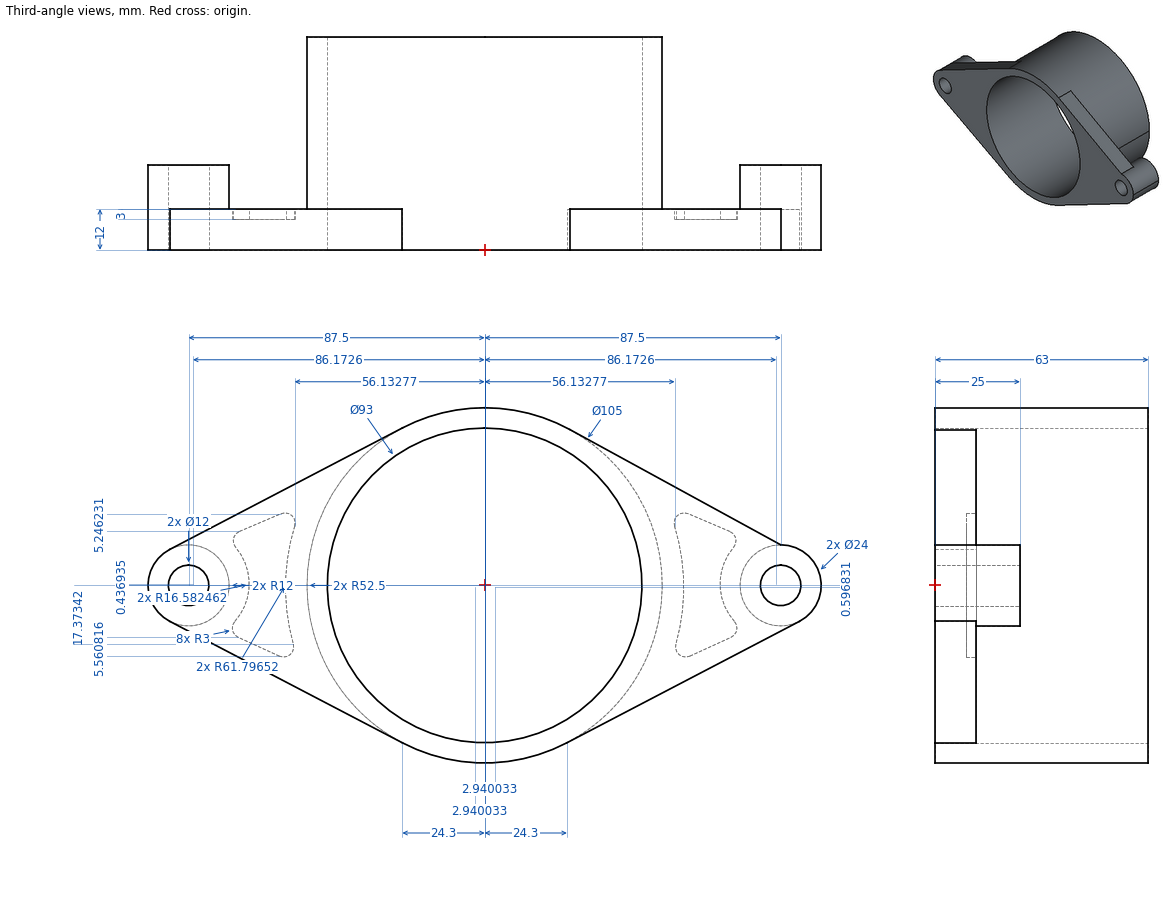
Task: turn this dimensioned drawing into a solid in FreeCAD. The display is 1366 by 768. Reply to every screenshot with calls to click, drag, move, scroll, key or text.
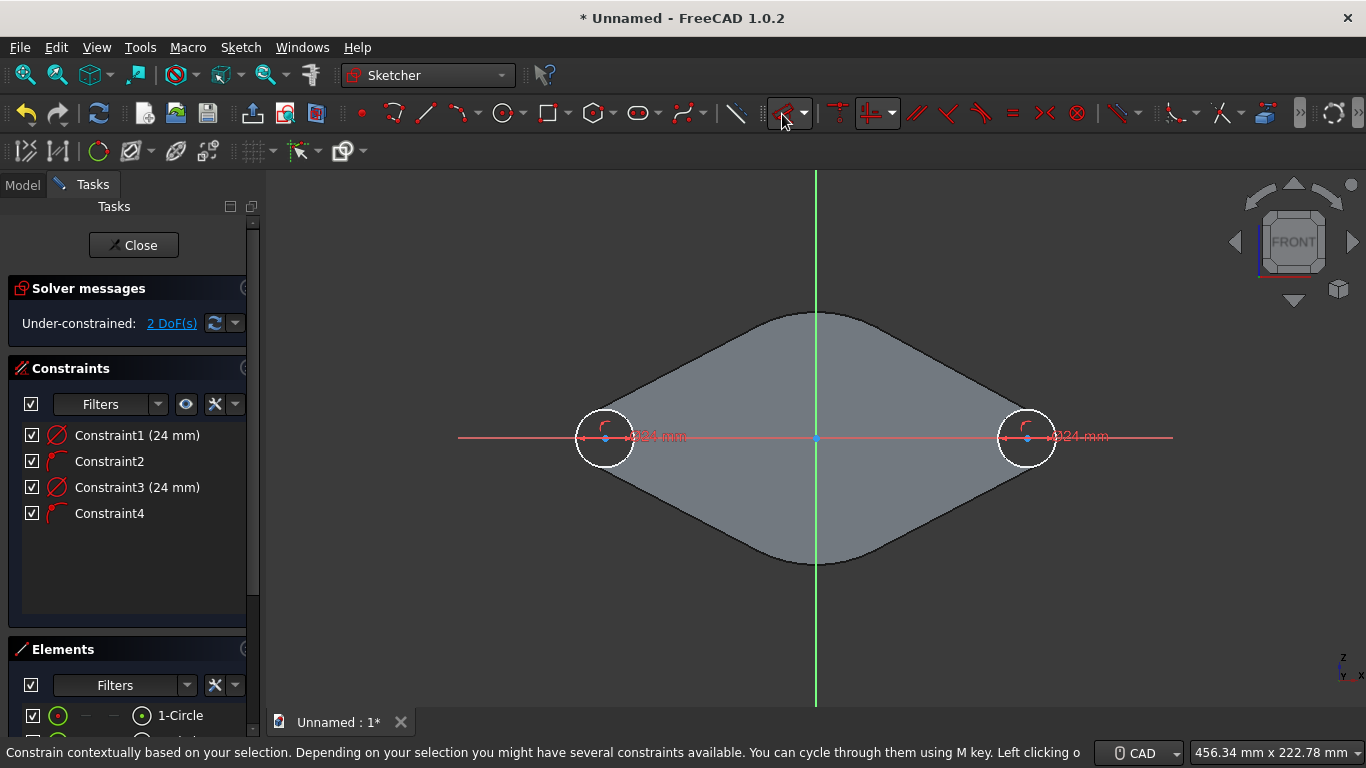
click(1027, 438)
click(921, 472)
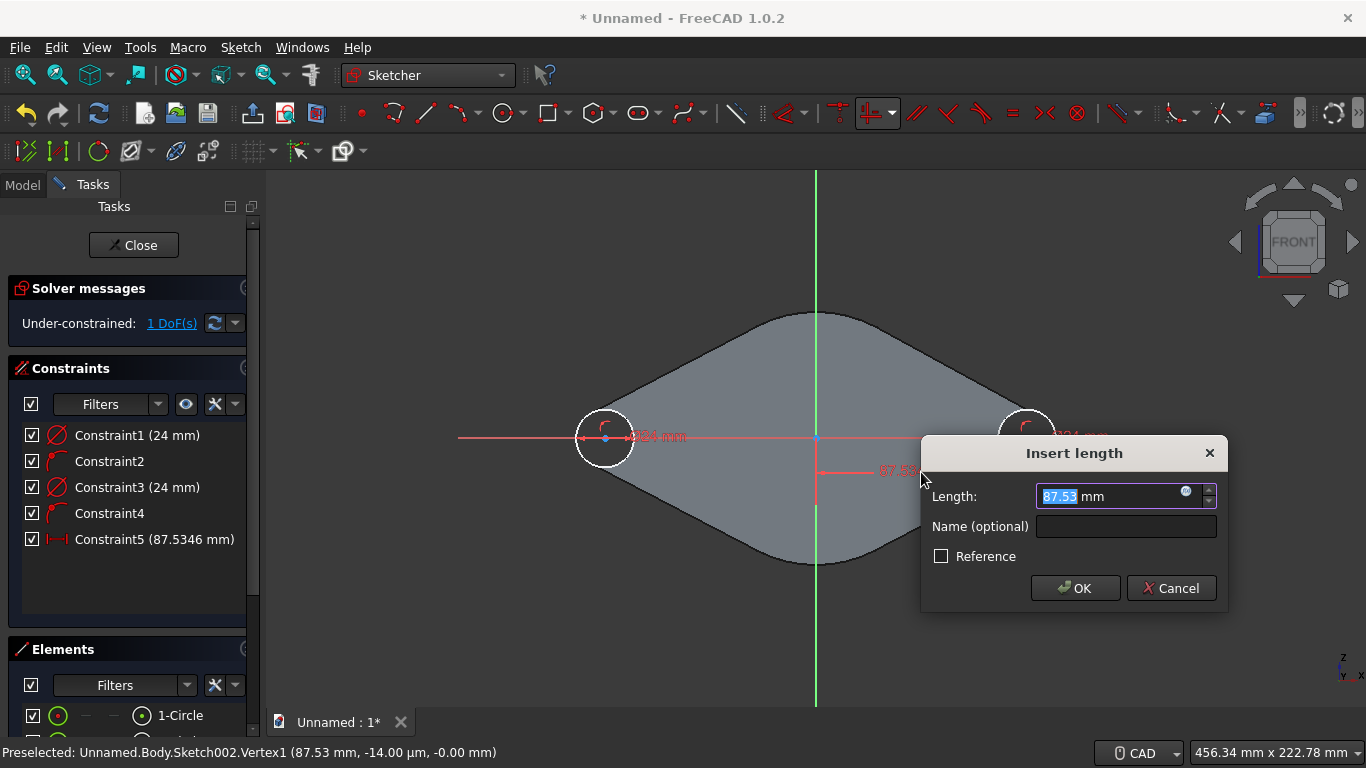
text(87.5)
key(Return)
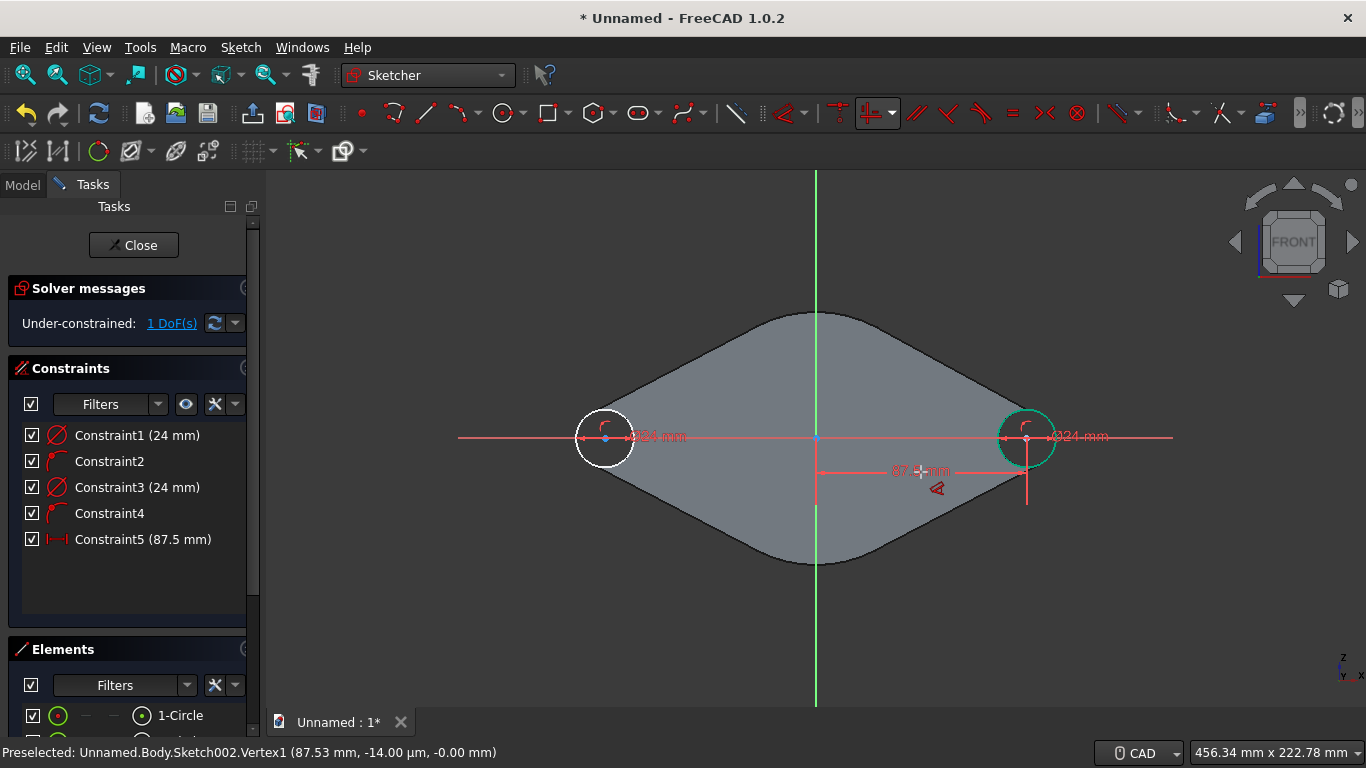
click(605, 438)
click(711, 472)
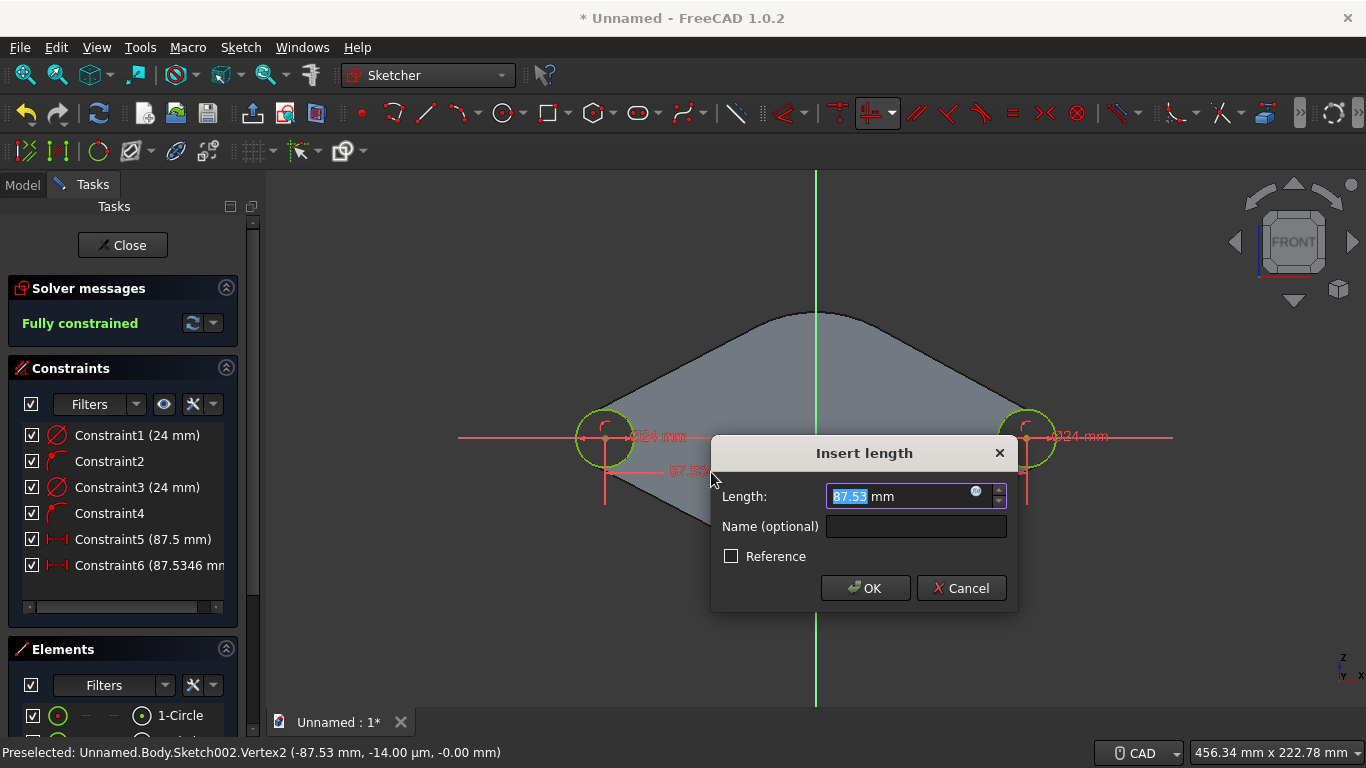
text(87.5)
key(Return)
key(Escape)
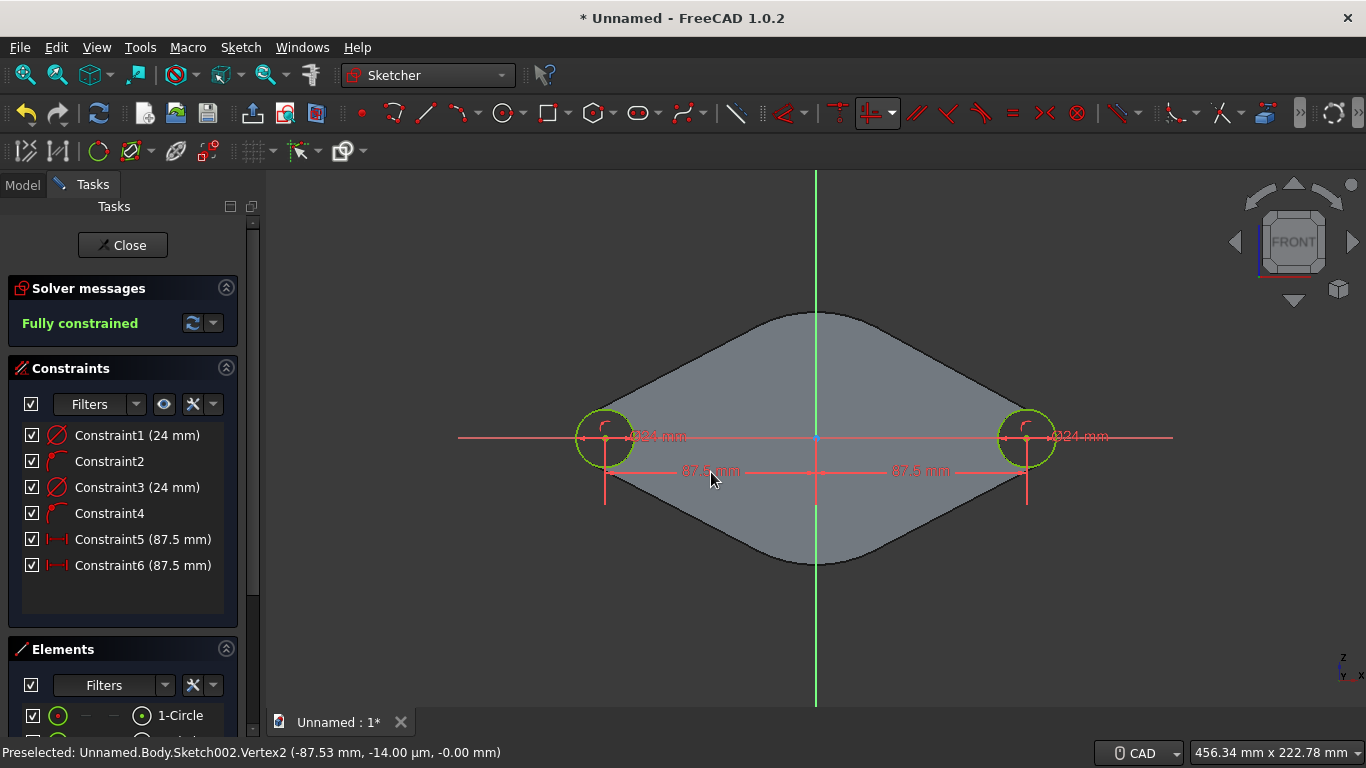
click(123, 245)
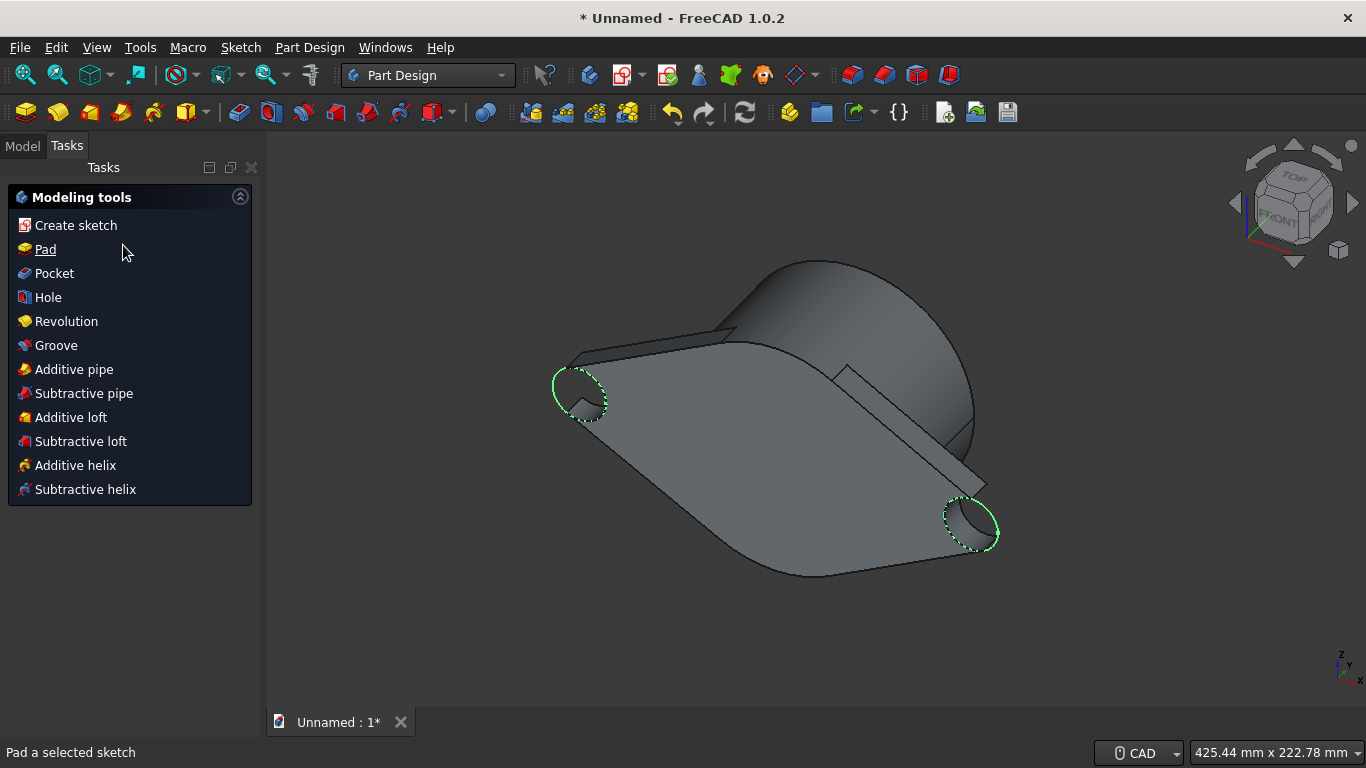
click(26, 112)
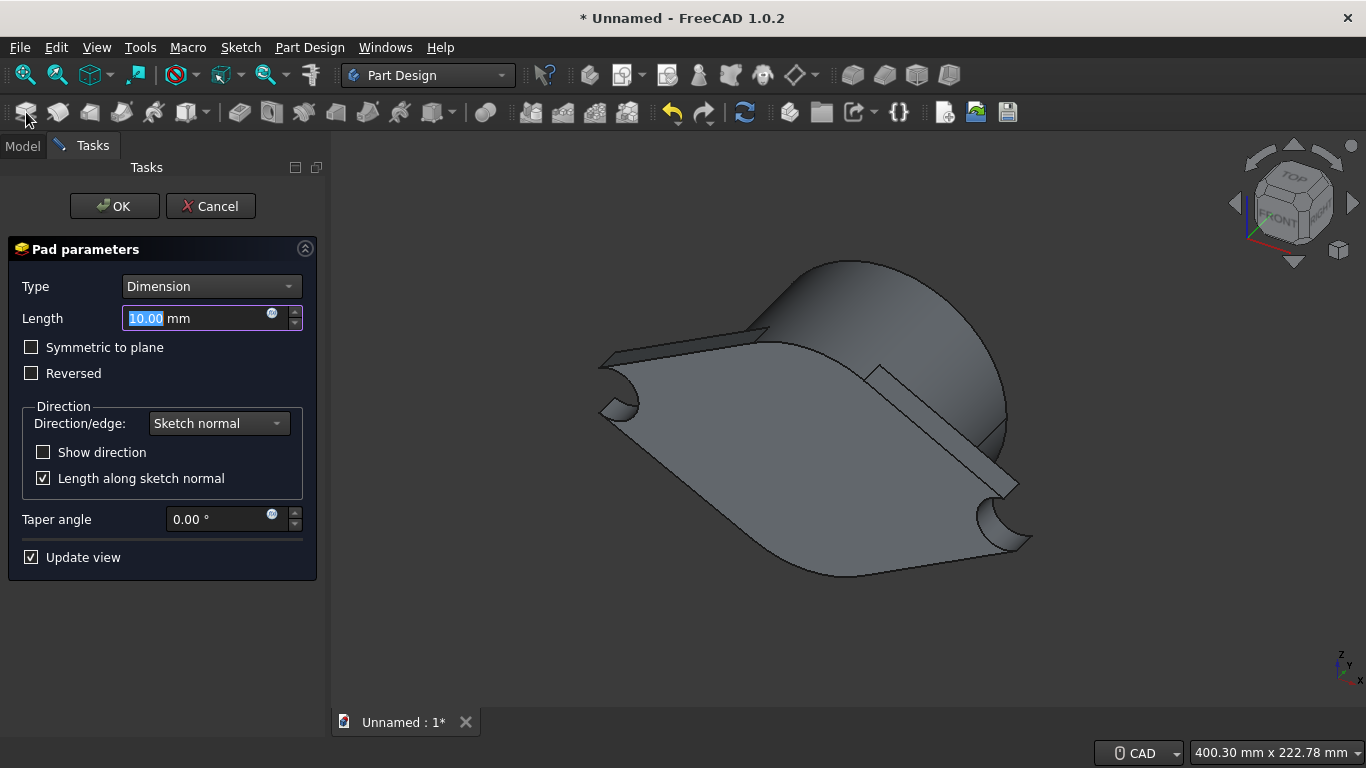
text(25)
key(Tab)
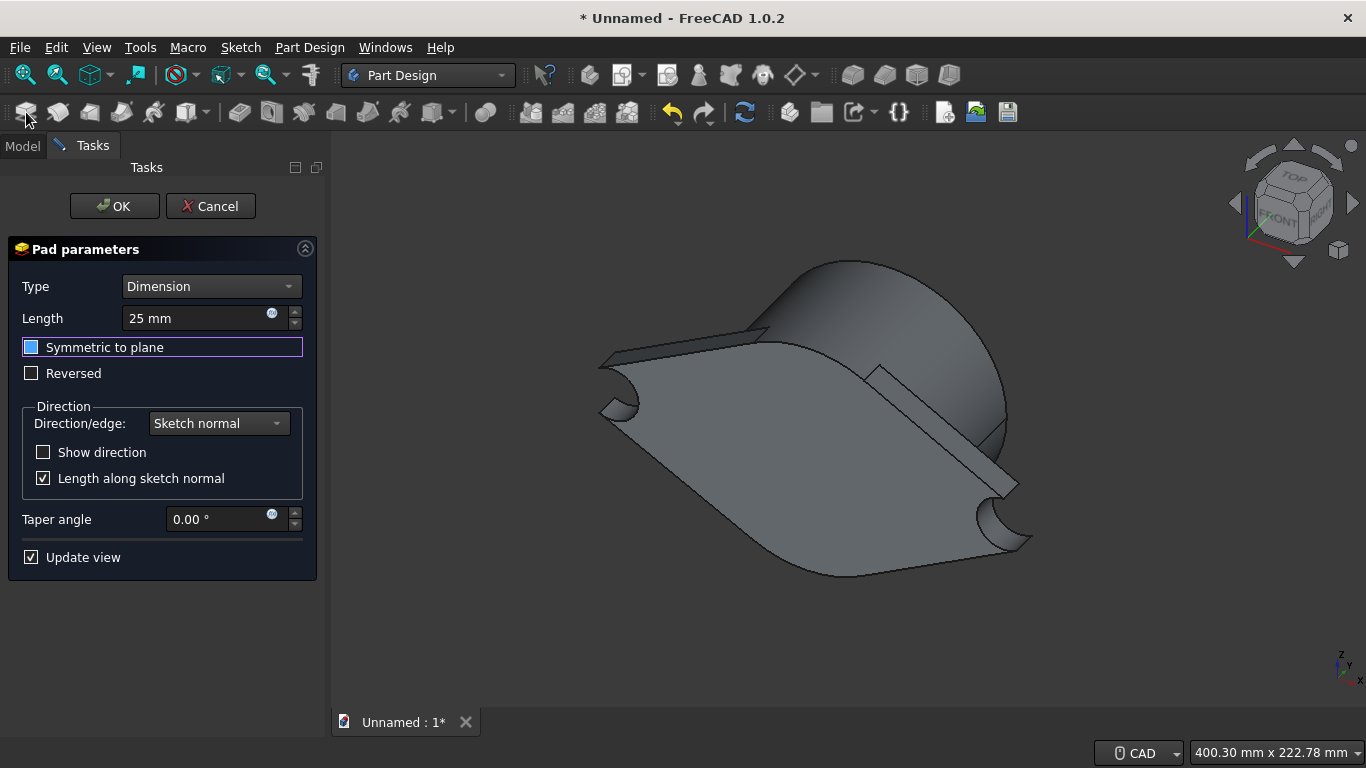
click(30, 373)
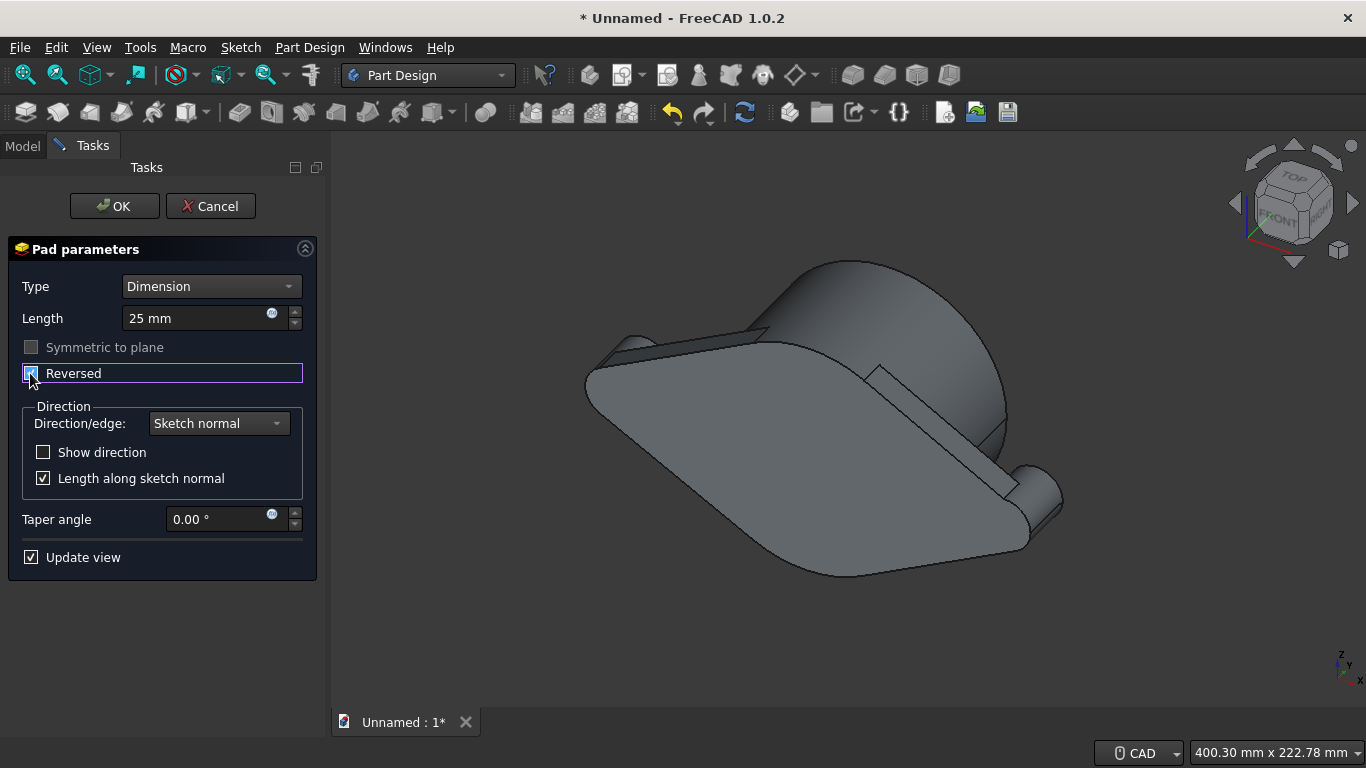
click(115, 206)